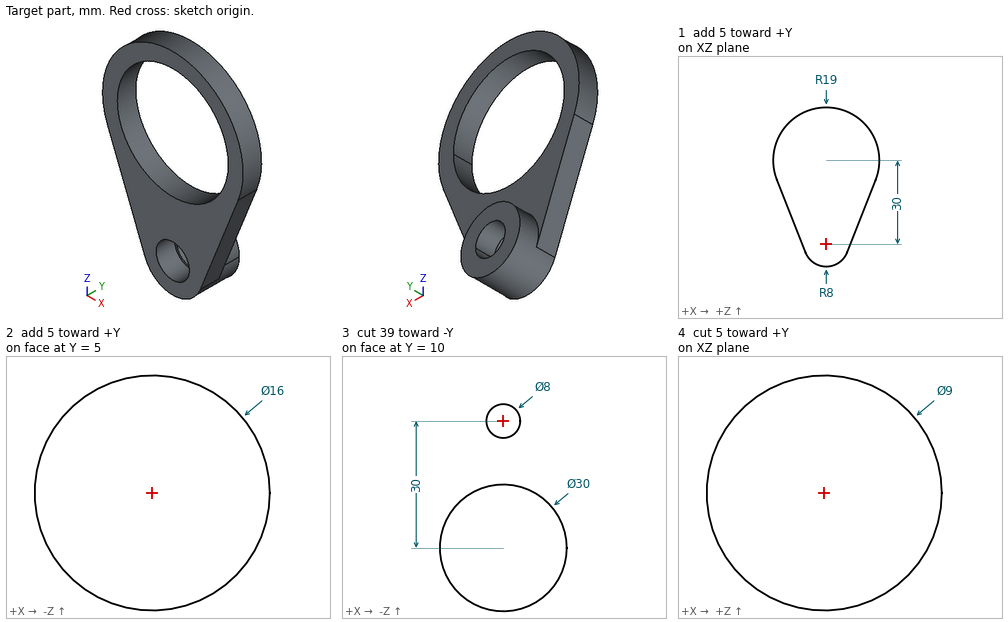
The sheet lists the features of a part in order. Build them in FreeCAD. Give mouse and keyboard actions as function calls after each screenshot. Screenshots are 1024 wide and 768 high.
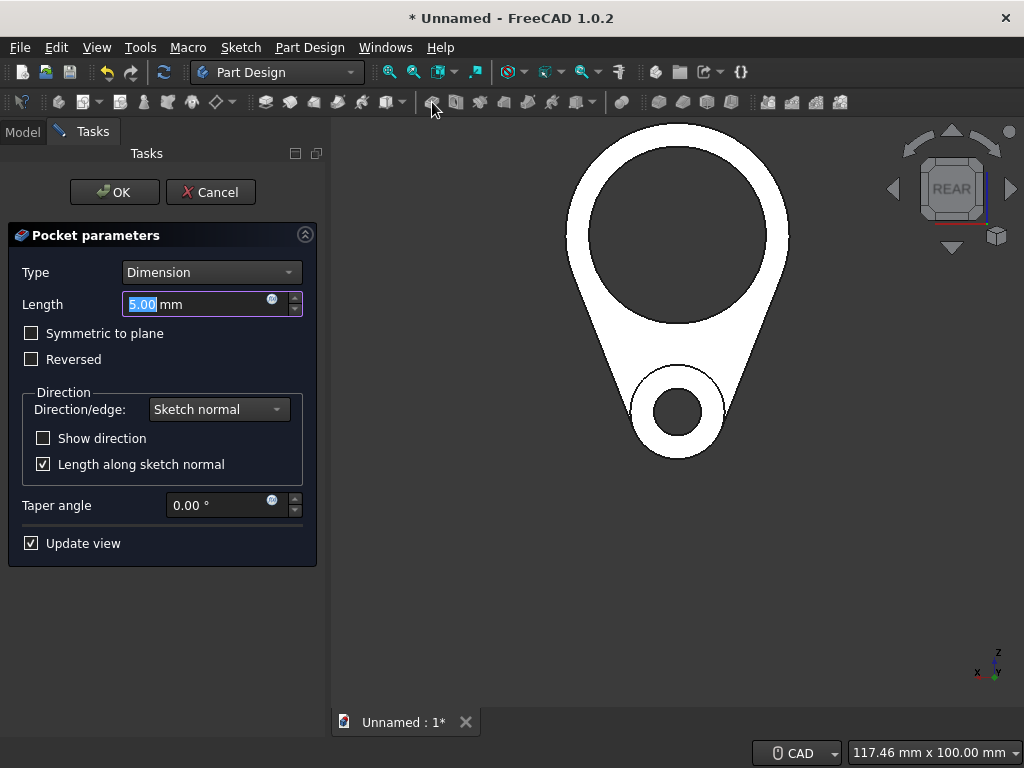
text(5)
key(Tab)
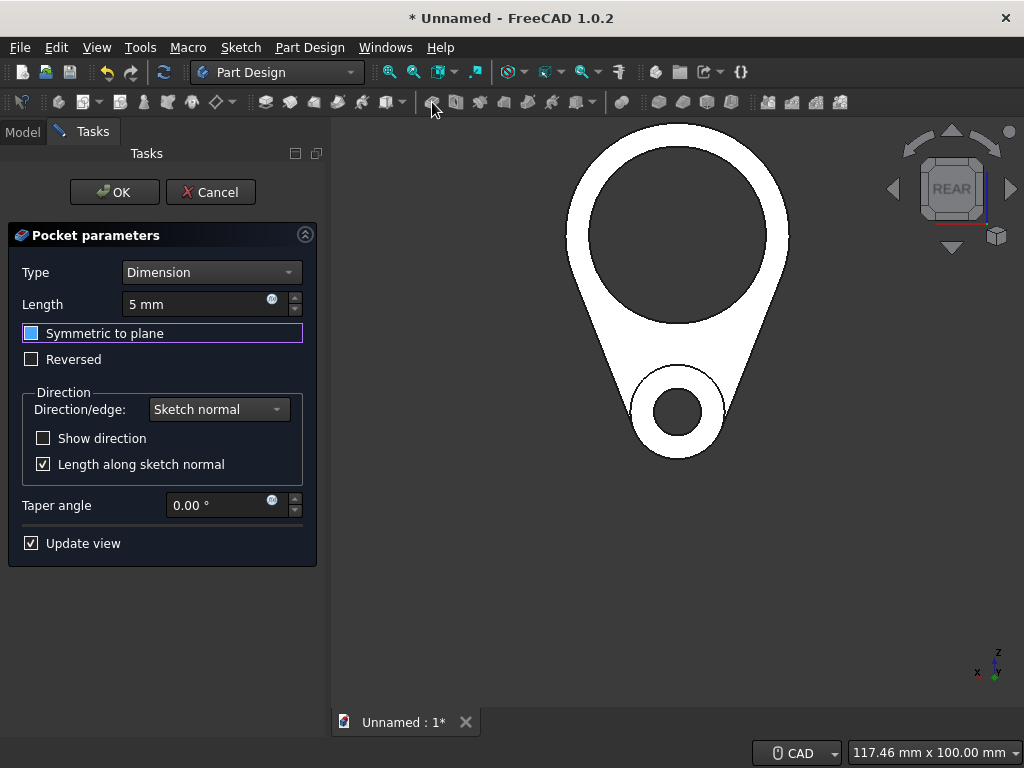
click(115, 192)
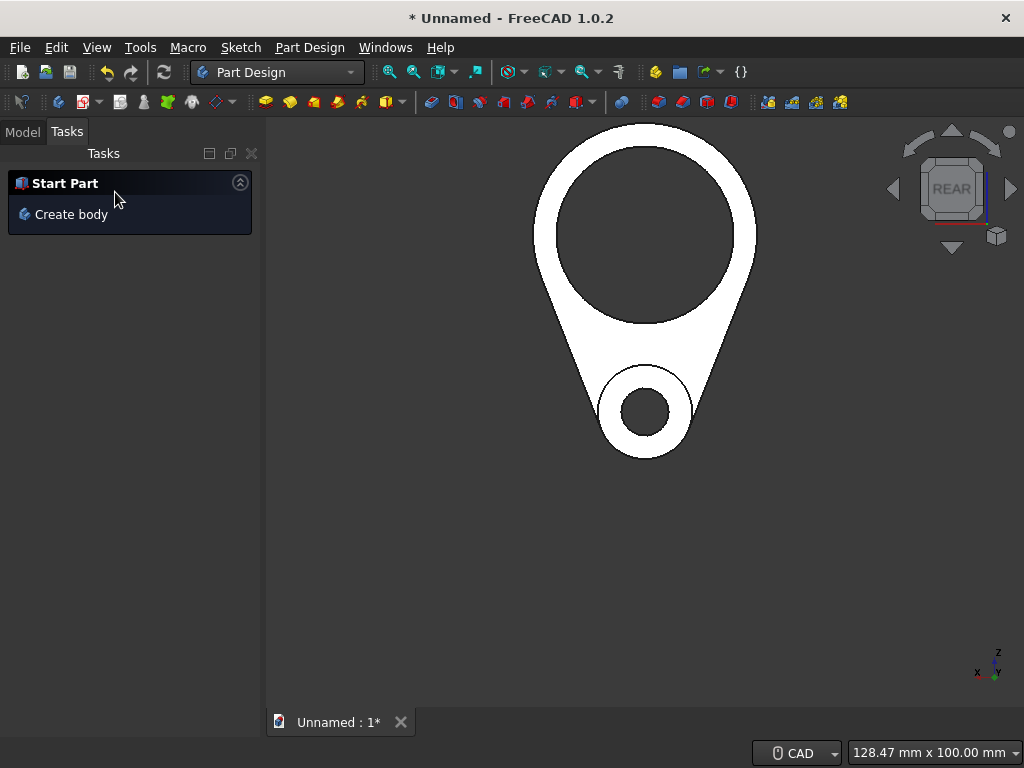
key(0)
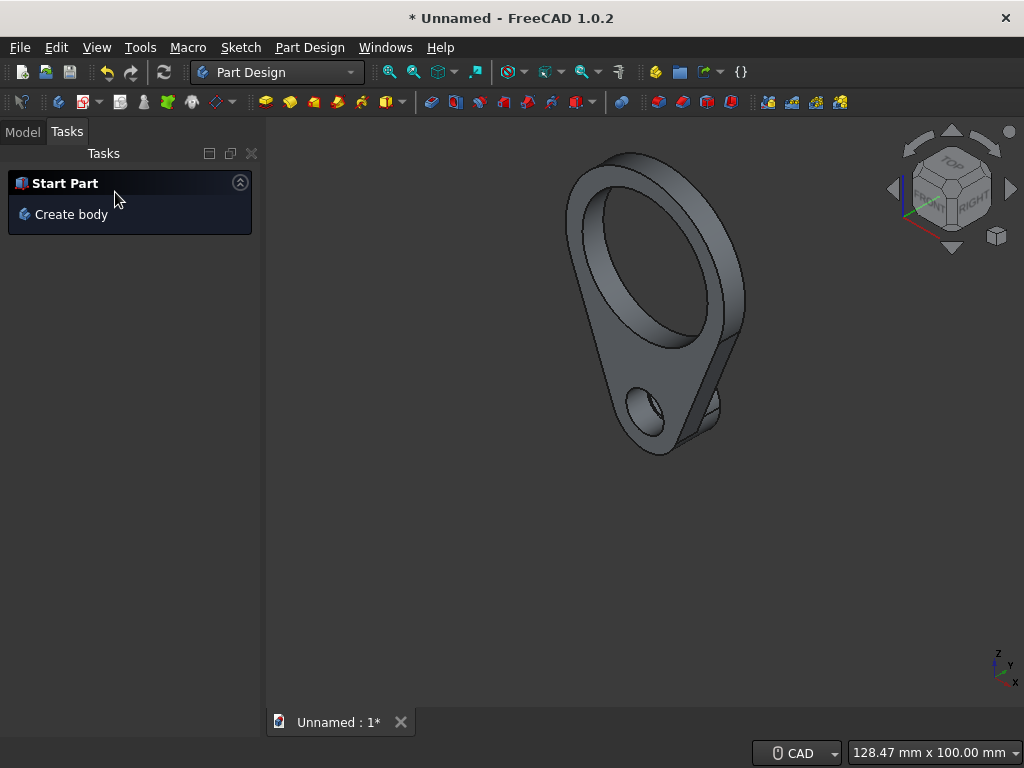
click(390, 72)